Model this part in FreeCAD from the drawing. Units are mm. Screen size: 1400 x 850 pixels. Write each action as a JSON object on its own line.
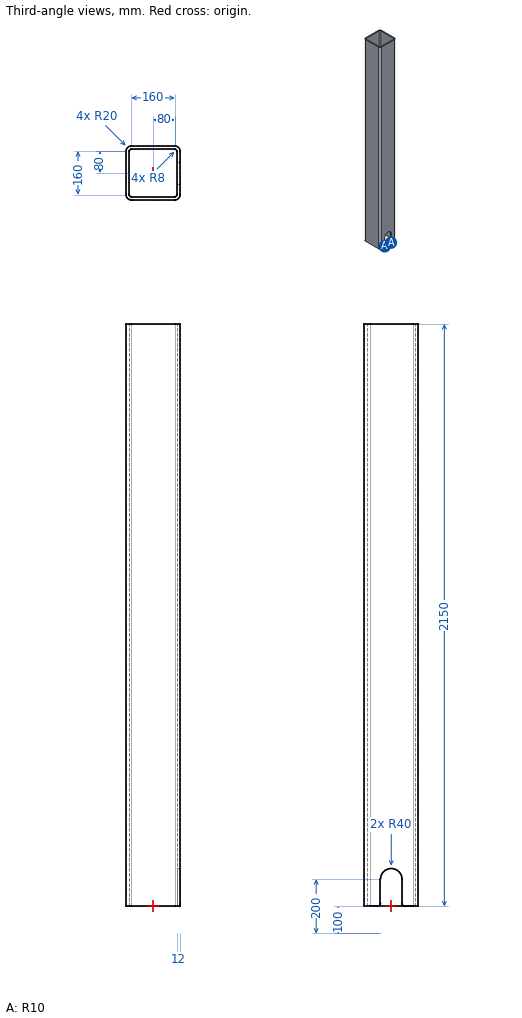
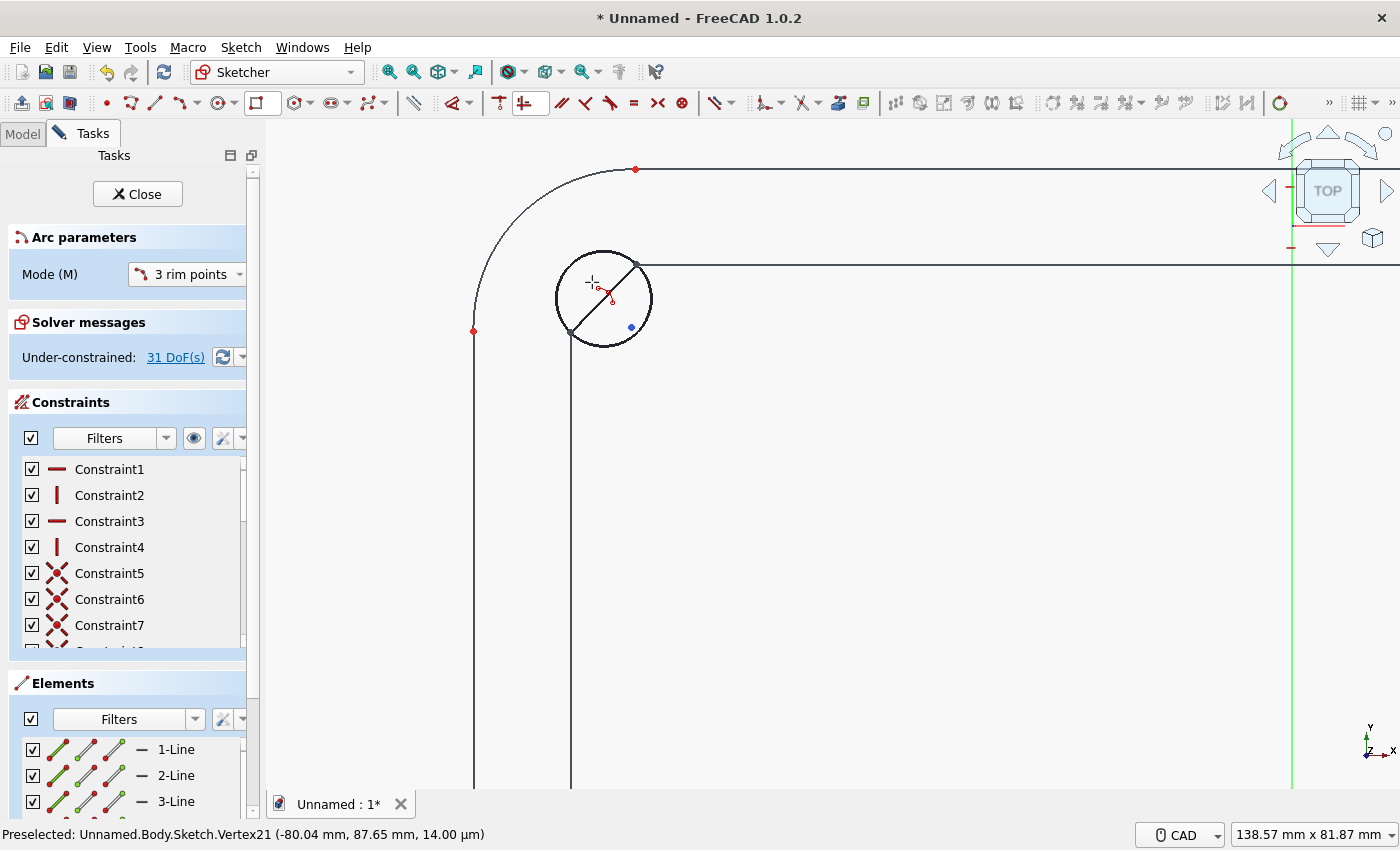
{"action": "left_click", "coordinate": [591, 281]}
{"action": "key", "text": "Escape"}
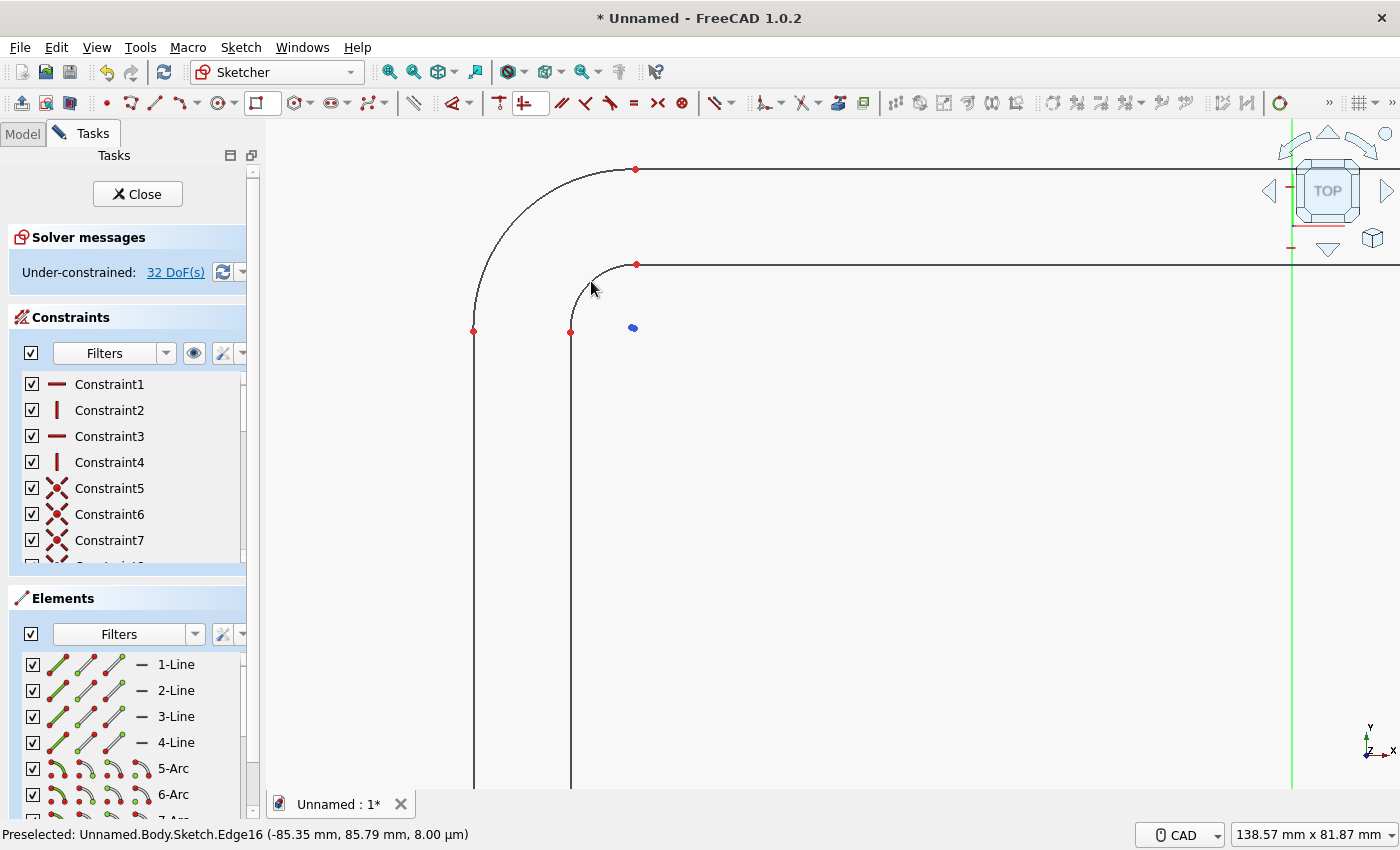
{"action": "scroll", "coordinate": [592, 281], "scroll_direction": "down", "scroll_amount": 7}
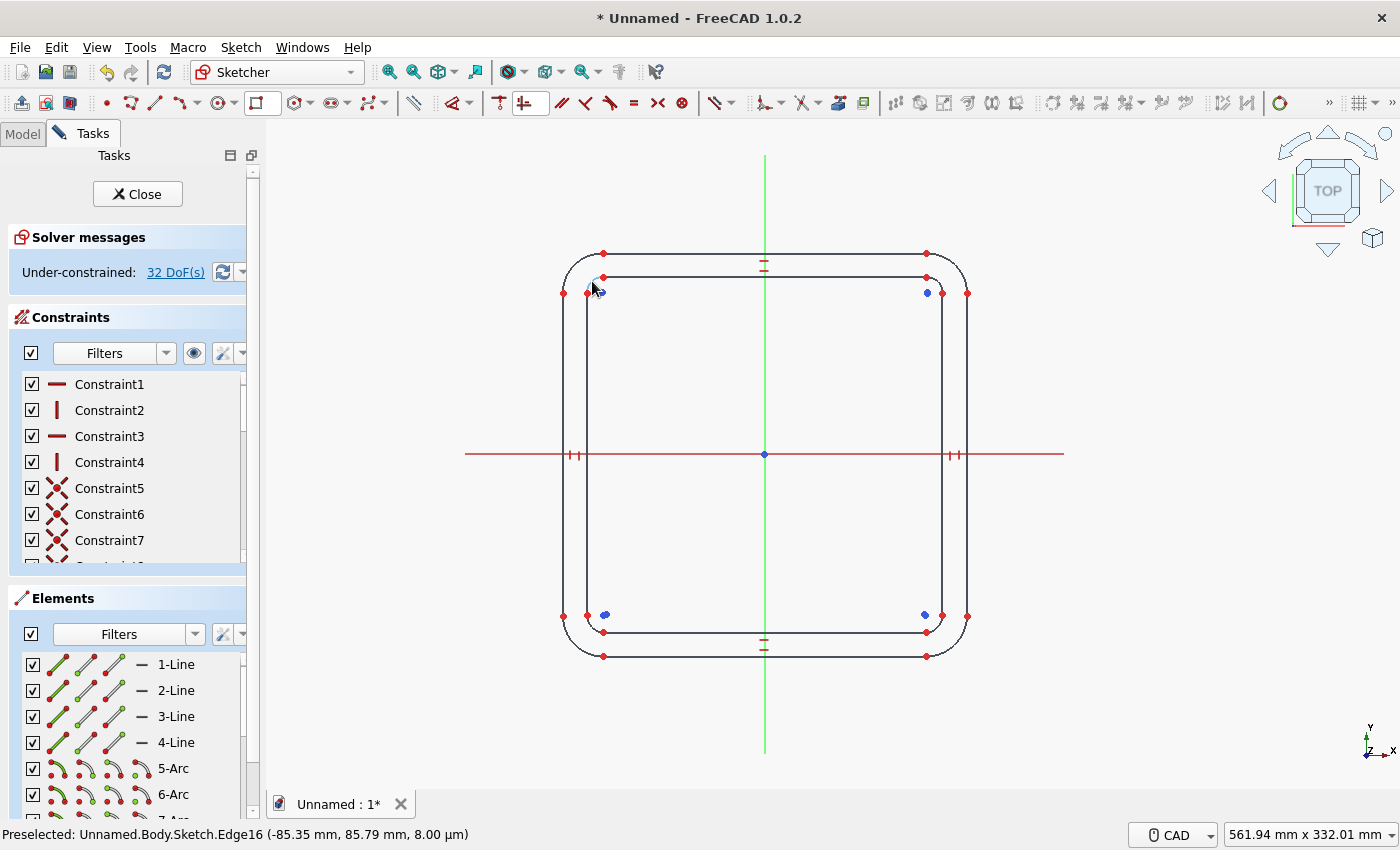
{"action": "left_click", "coordinate": [700, 254]}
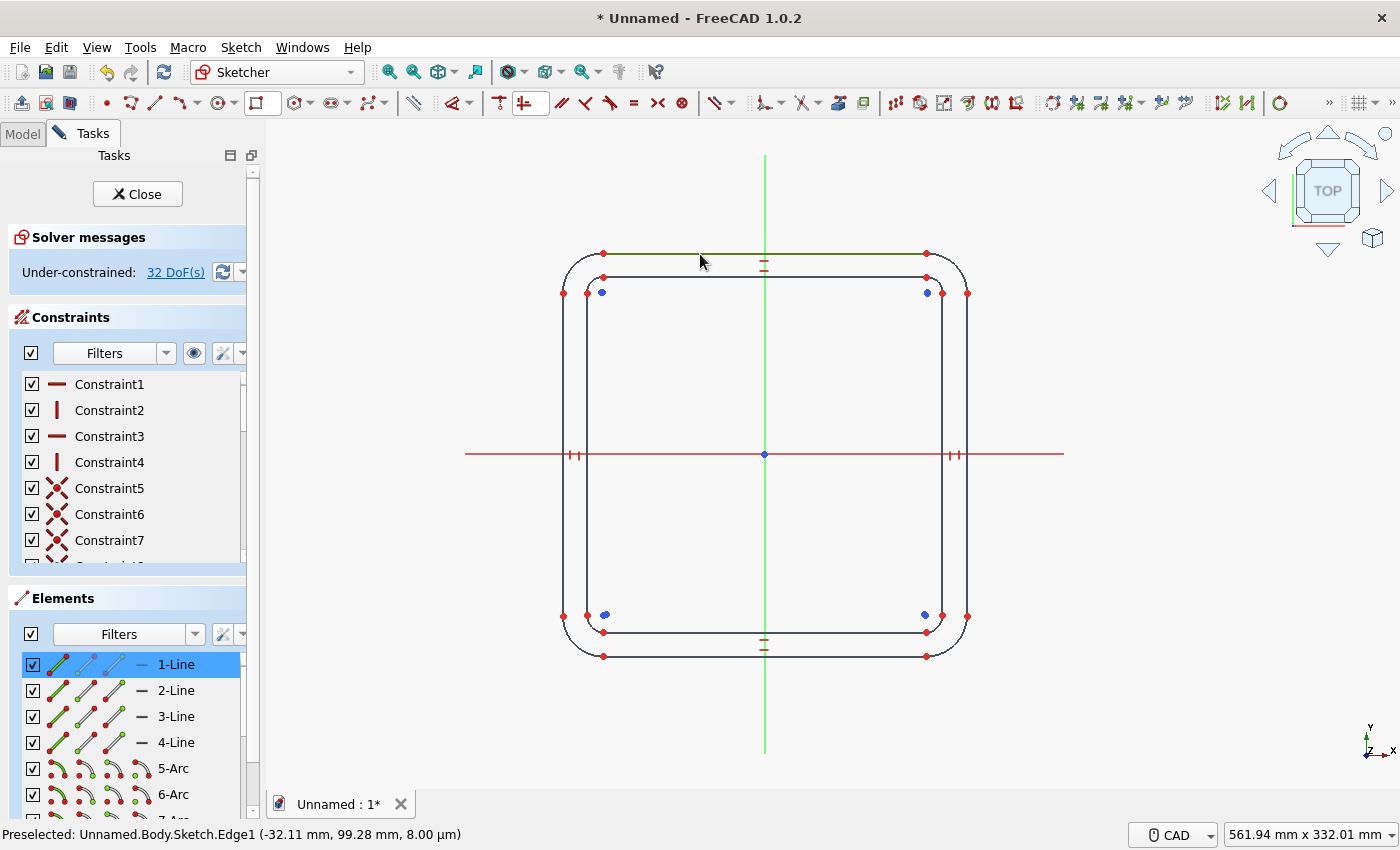
{"action": "left_click", "coordinate": [585, 258]}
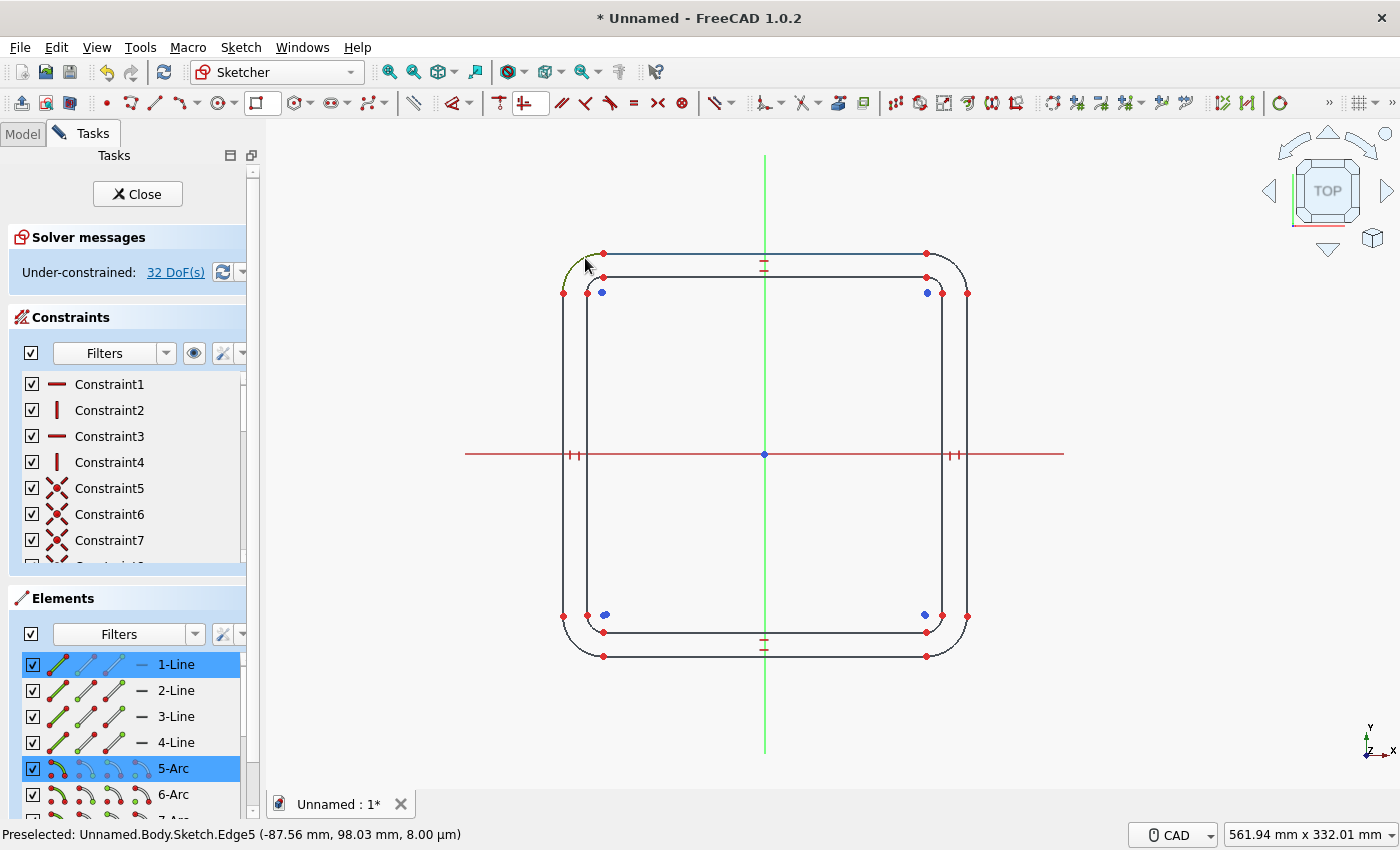
{"action": "left_click", "coordinate": [610, 104]}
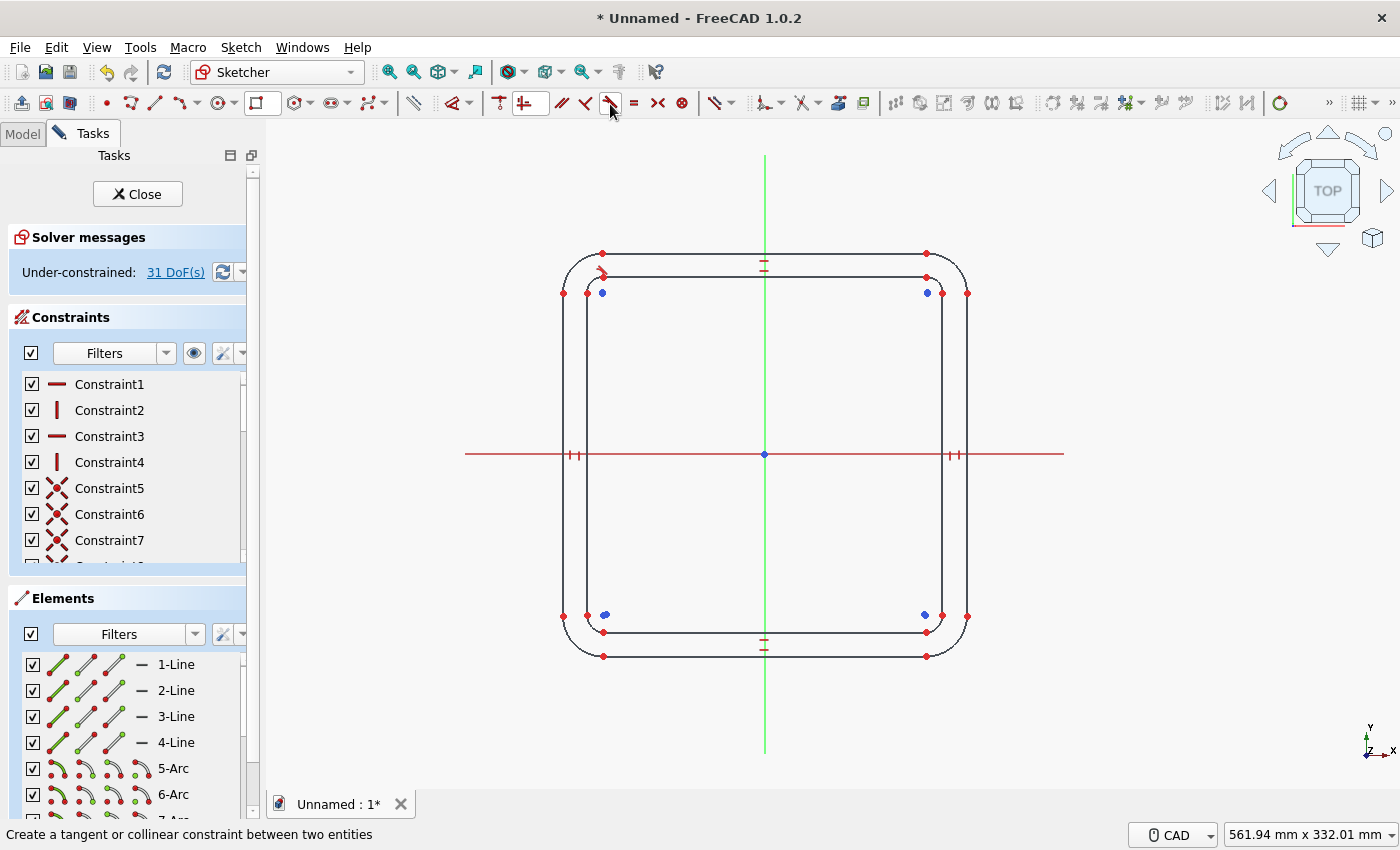
{"action": "left_click", "coordinate": [829, 254]}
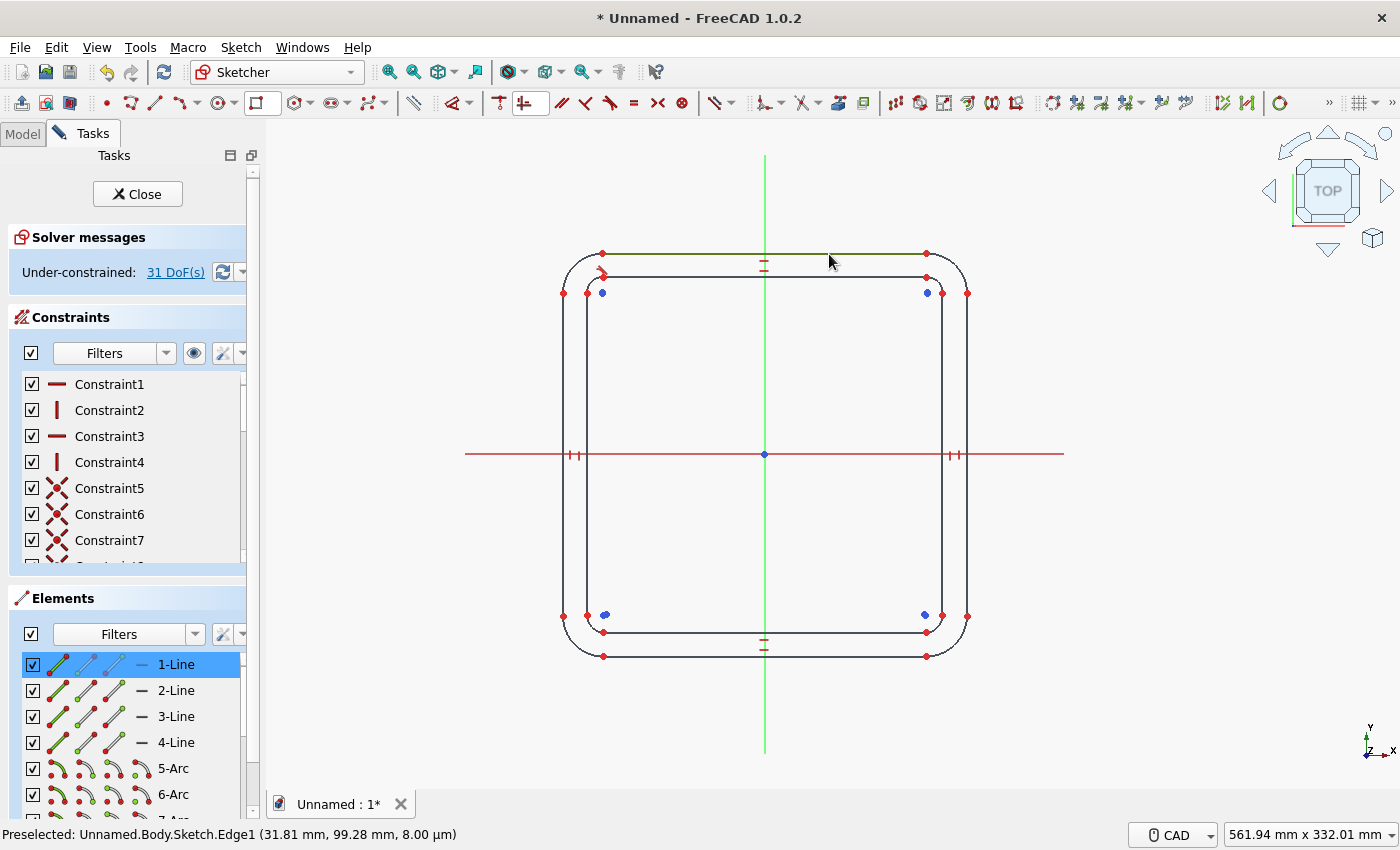
{"action": "left_click", "coordinate": [963, 275]}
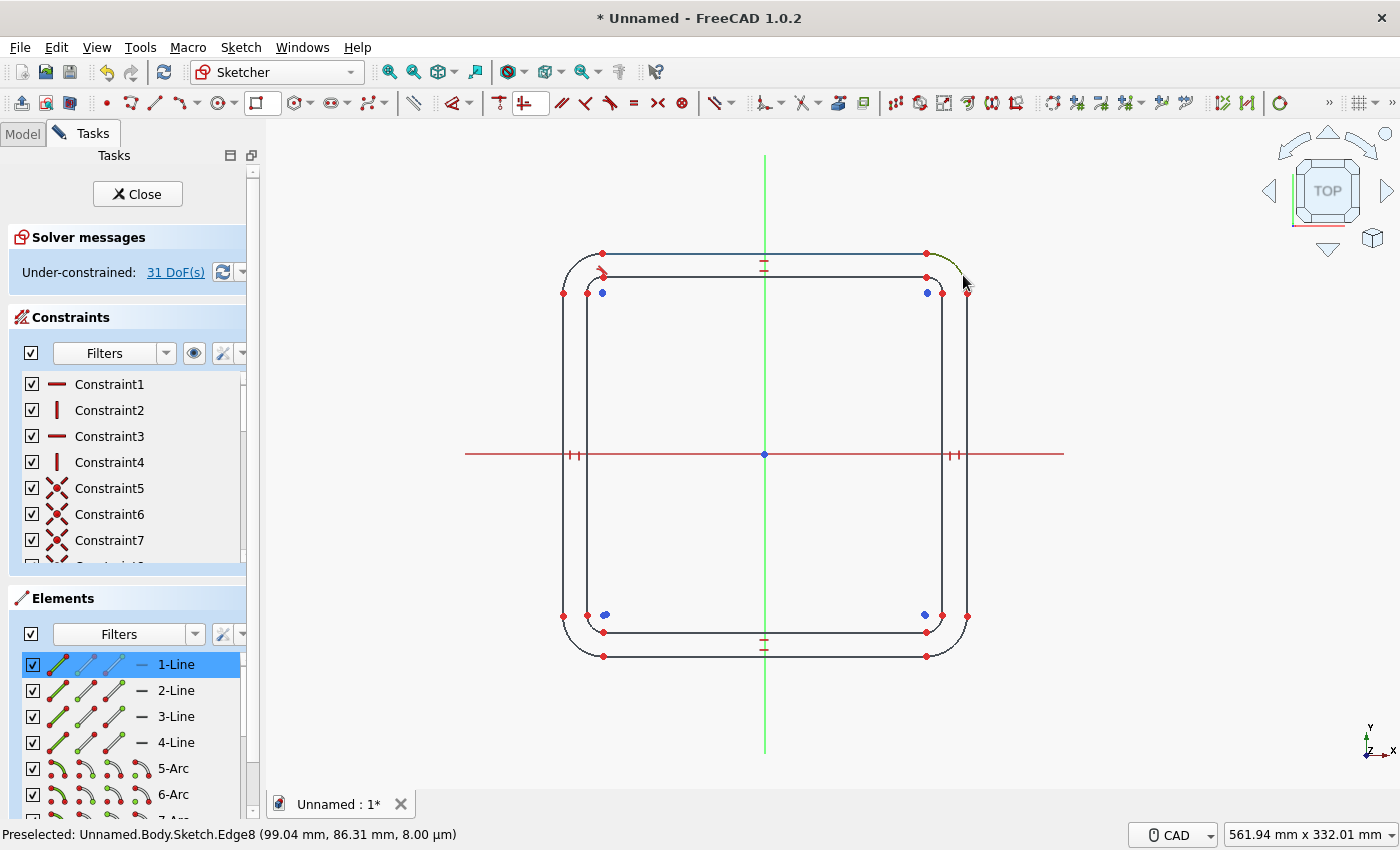
{"action": "left_click", "coordinate": [610, 104]}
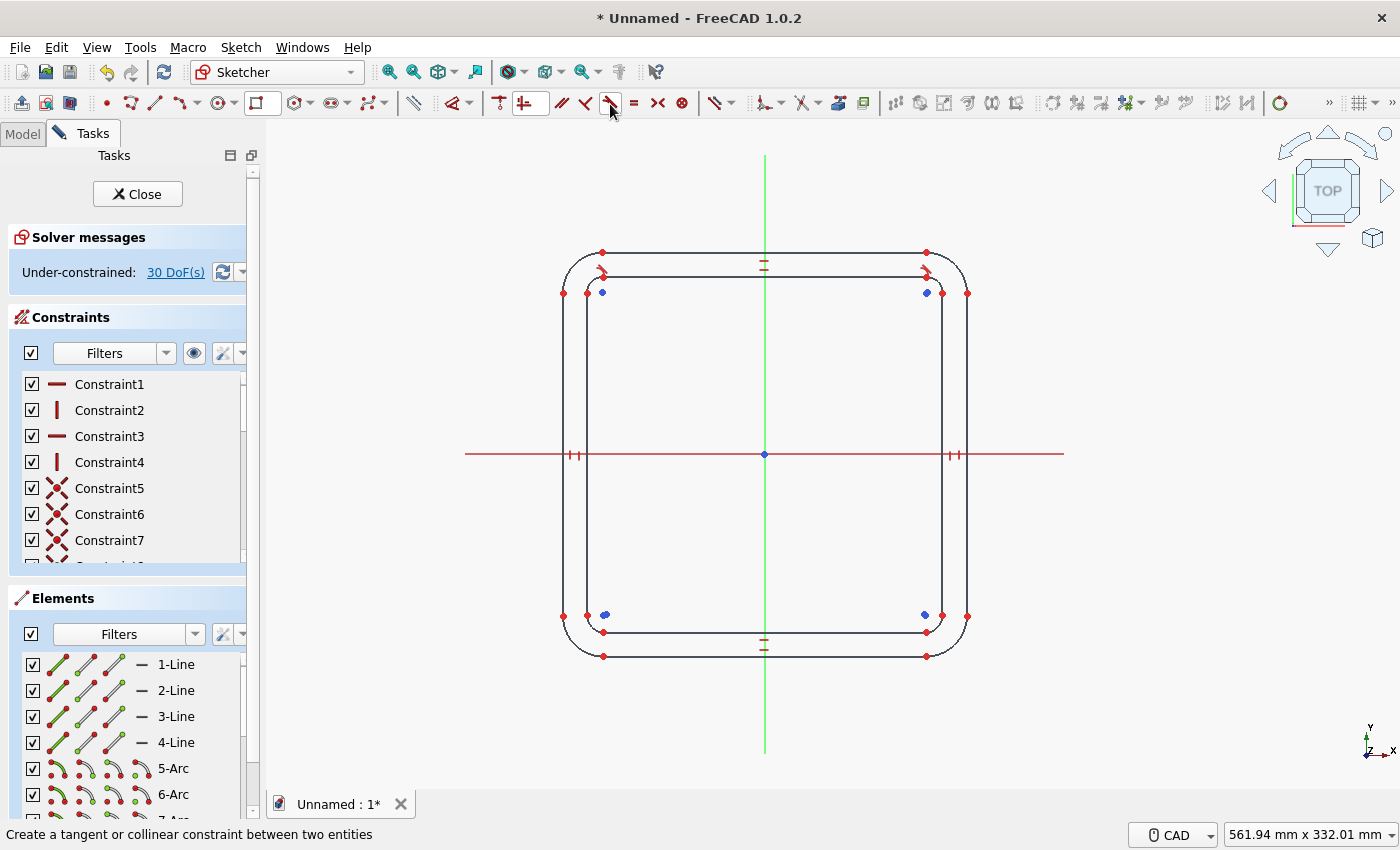
{"action": "left_click", "coordinate": [563, 391]}